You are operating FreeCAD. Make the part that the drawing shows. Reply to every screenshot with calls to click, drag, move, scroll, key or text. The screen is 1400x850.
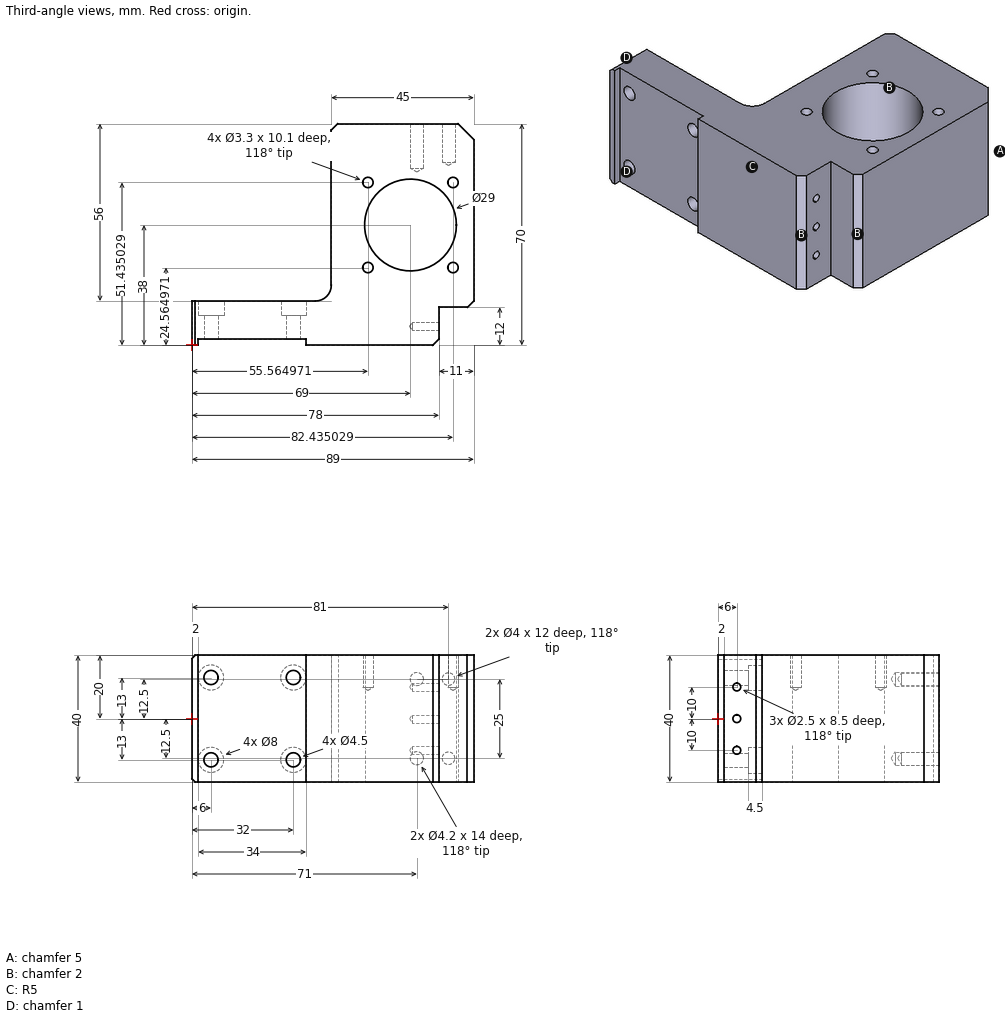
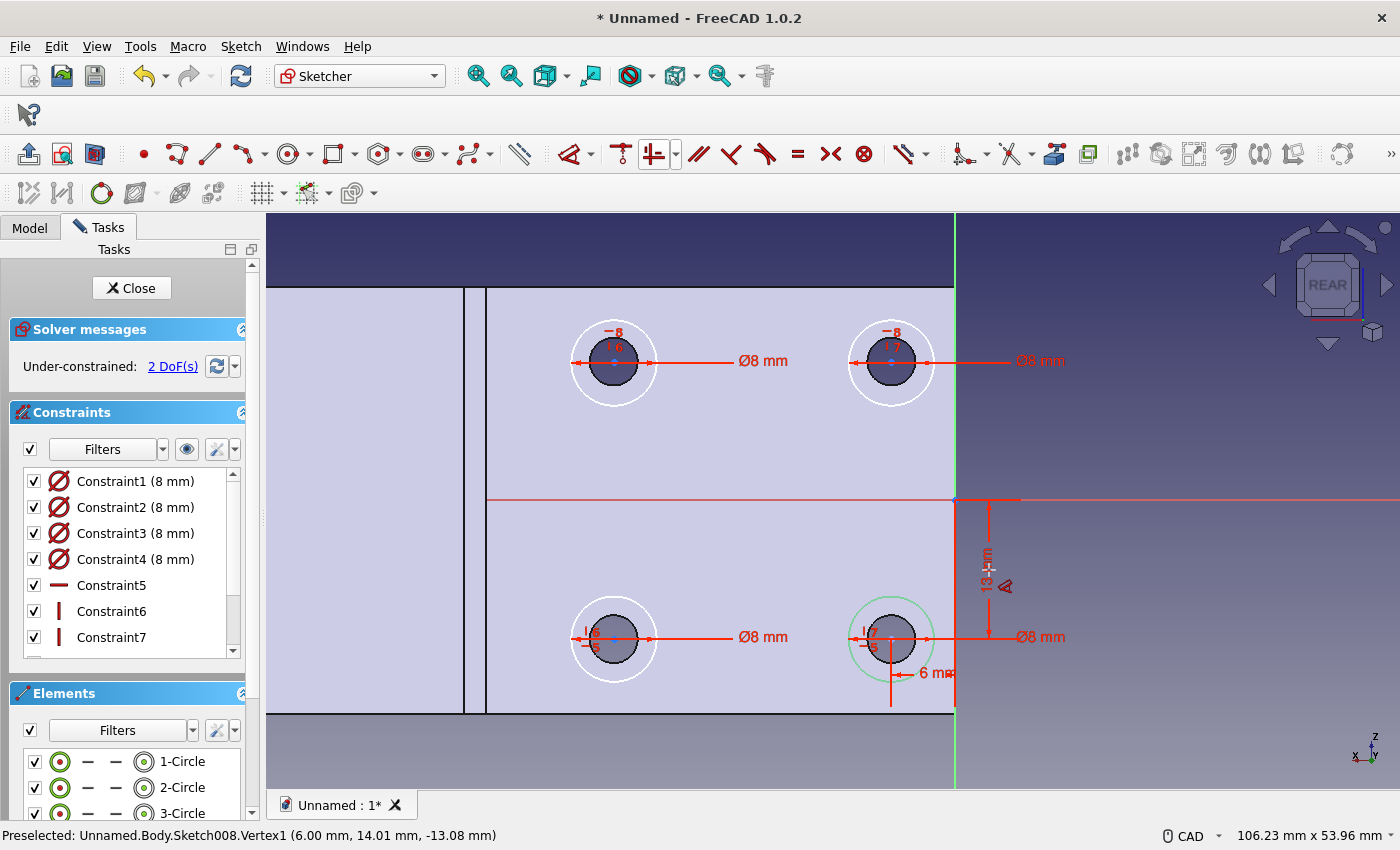
click(614, 639)
click(785, 673)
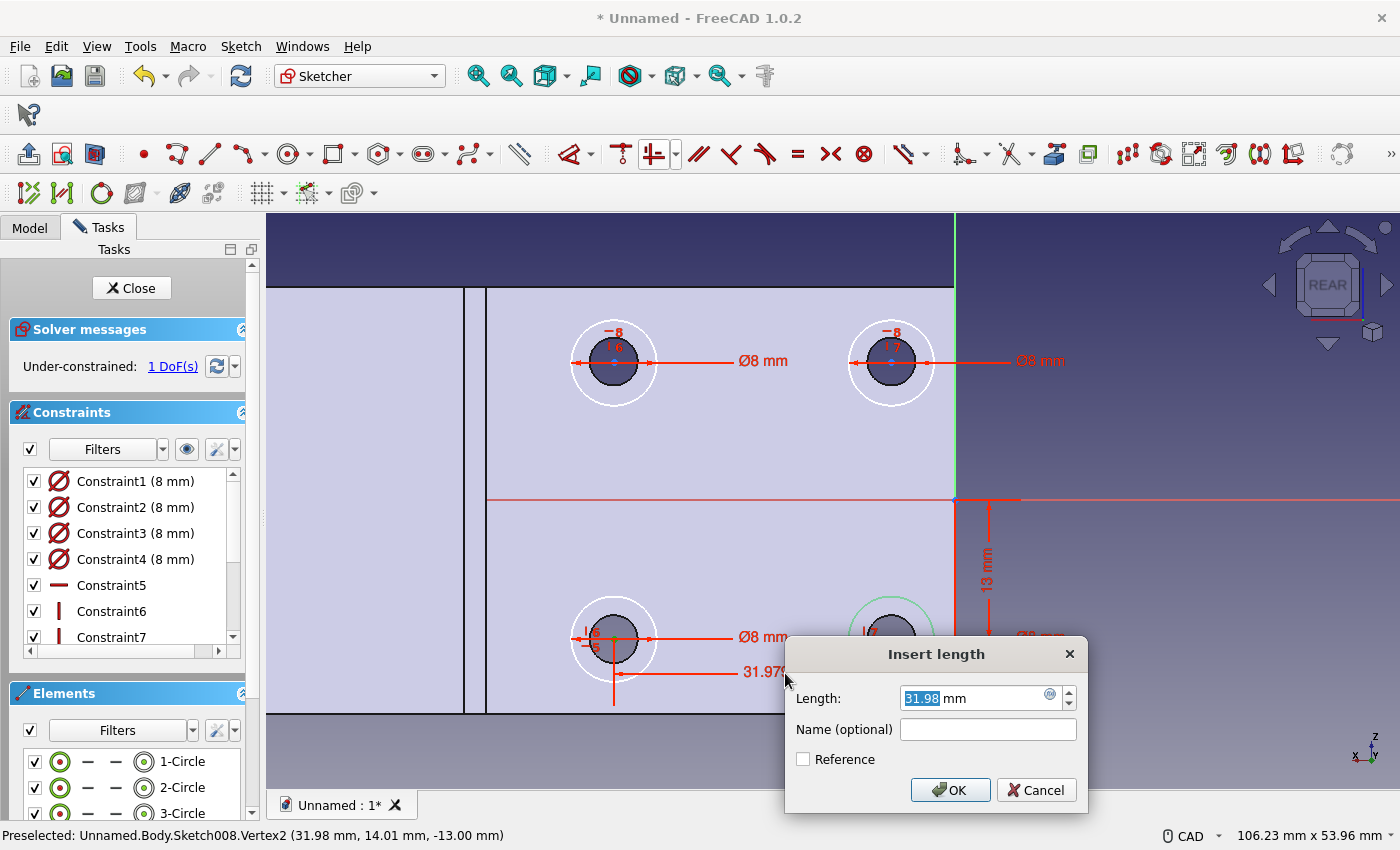
text(32)
key(Return)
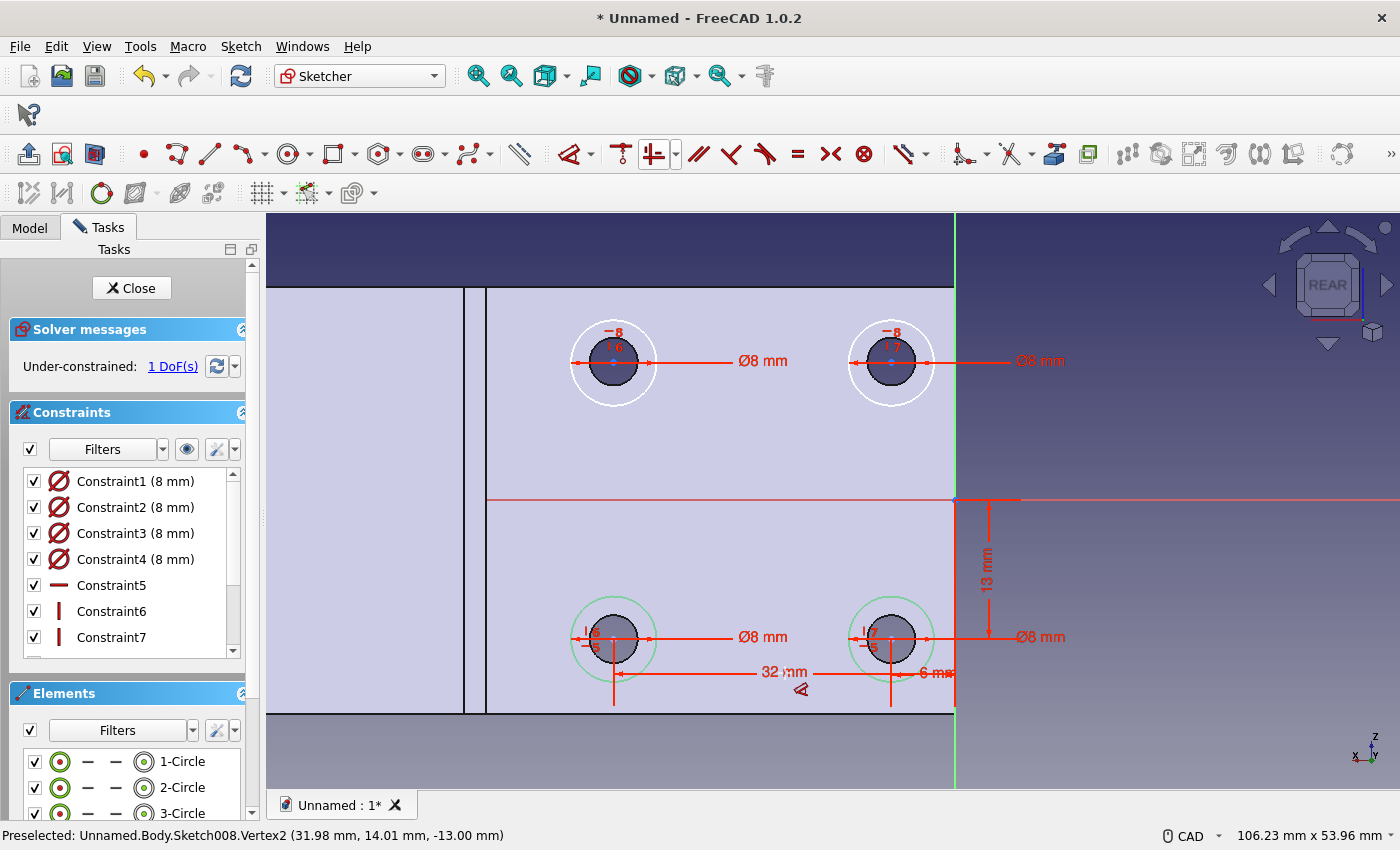
click(614, 363)
click(989, 432)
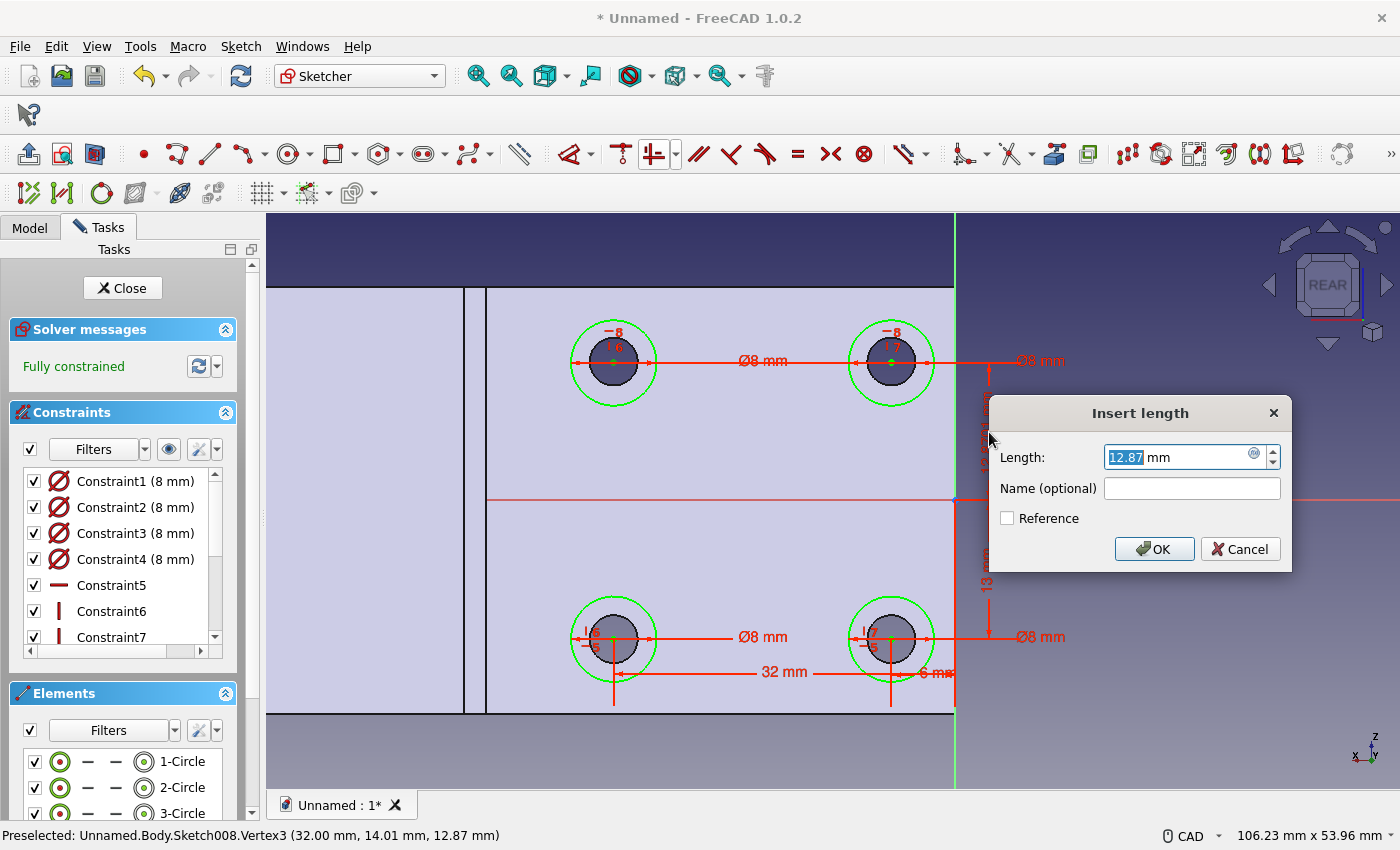
text(13)
key(Return)
key(Escape)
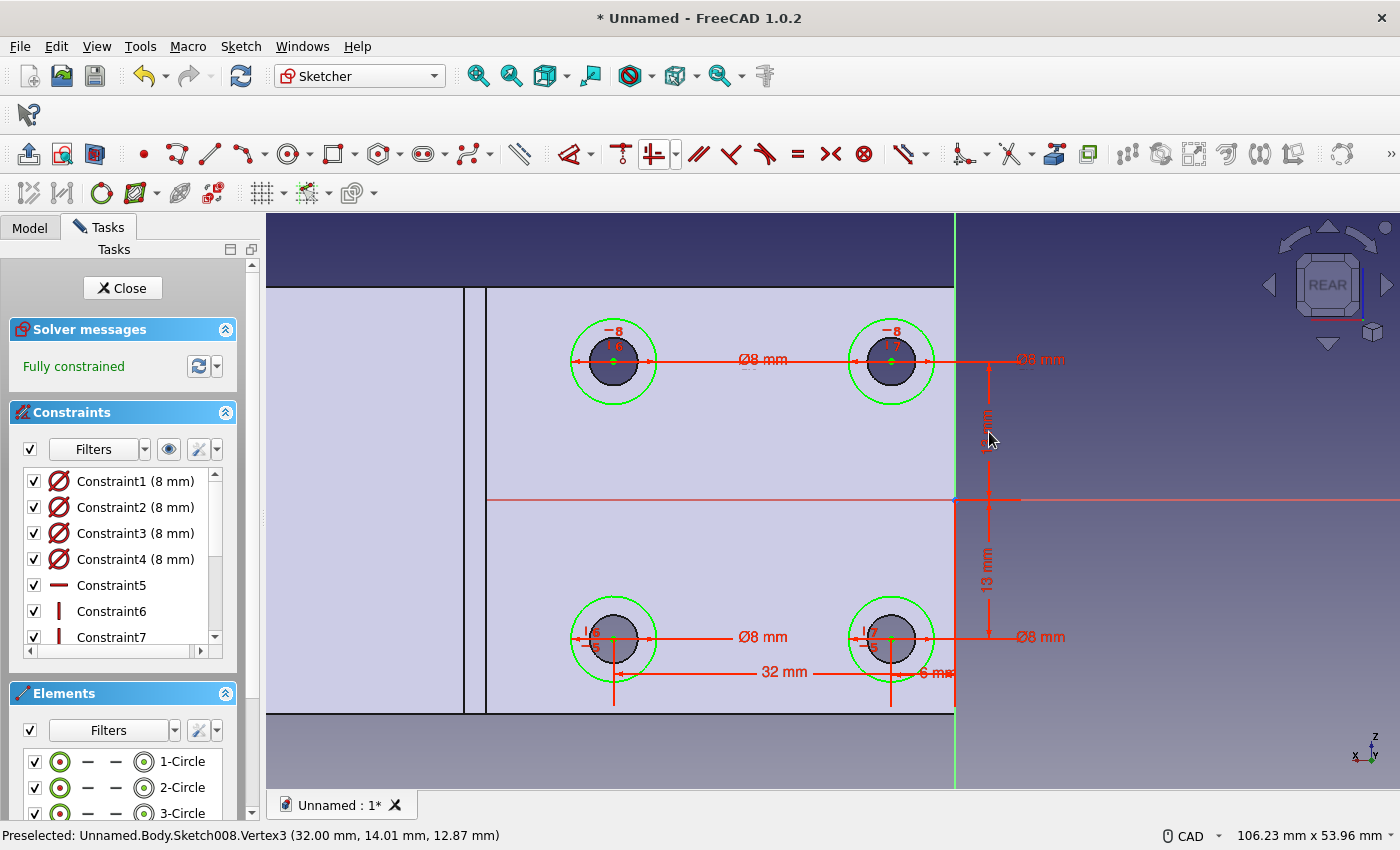
click(123, 288)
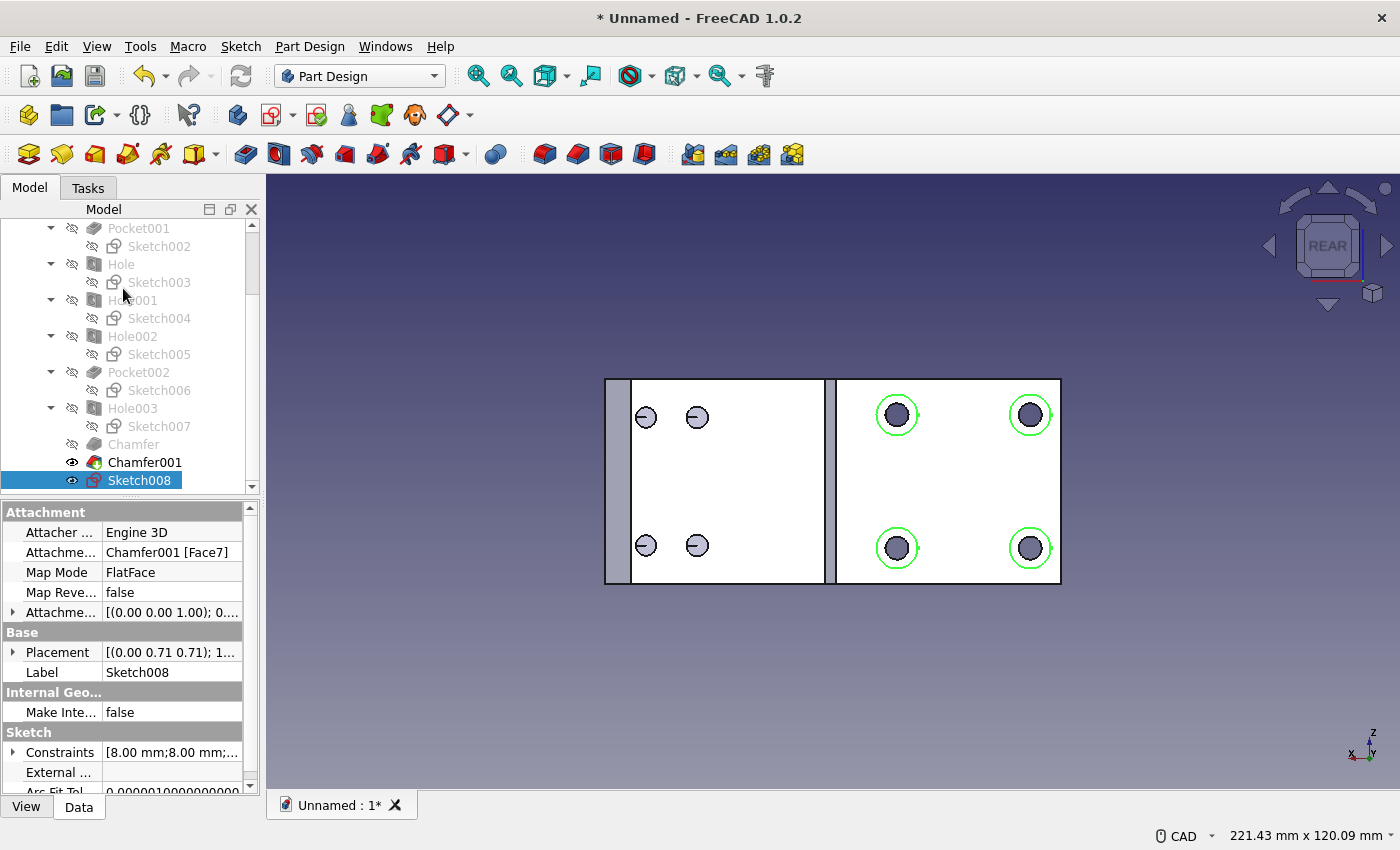
click(246, 154)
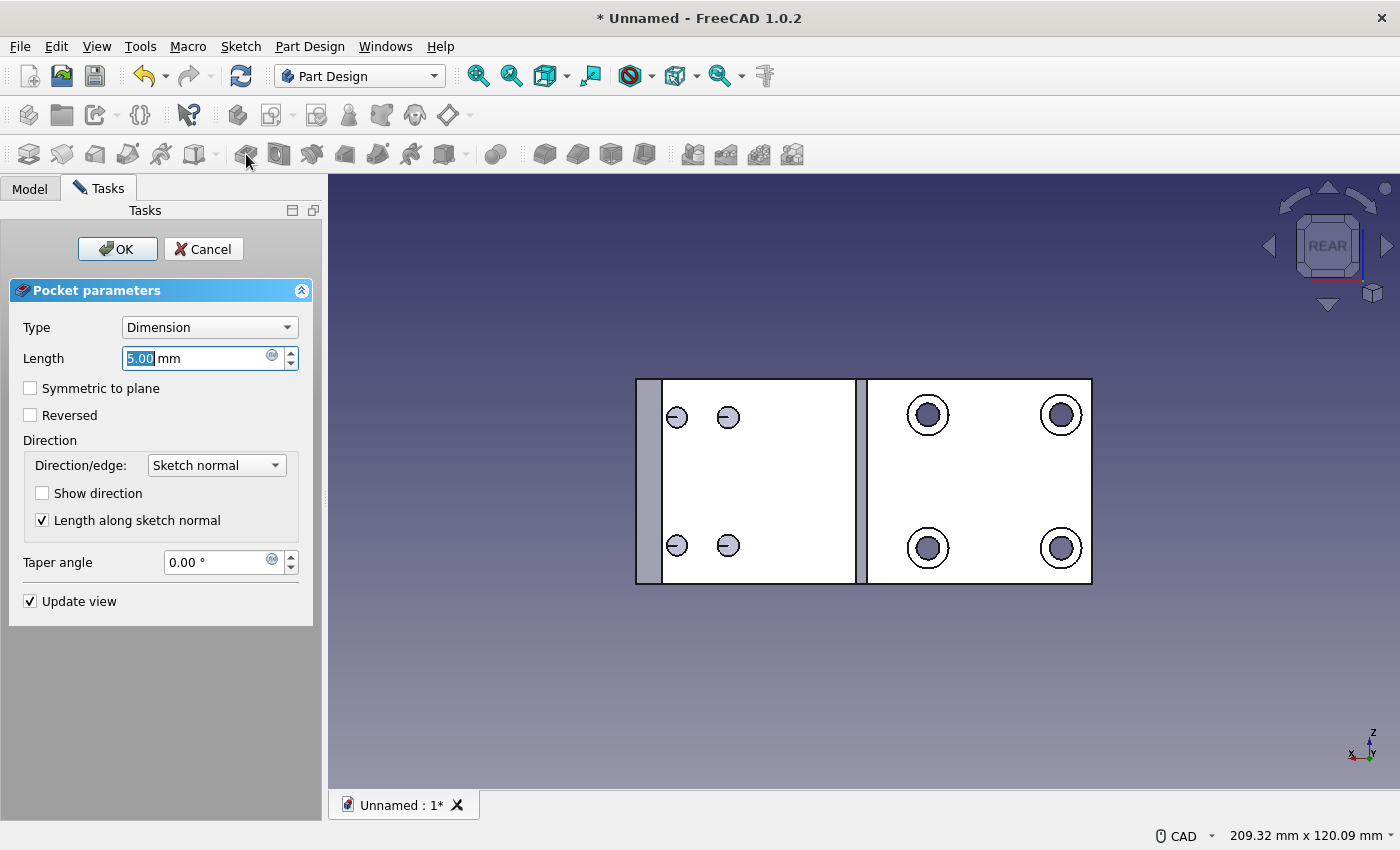
text(4.5)
key(Tab)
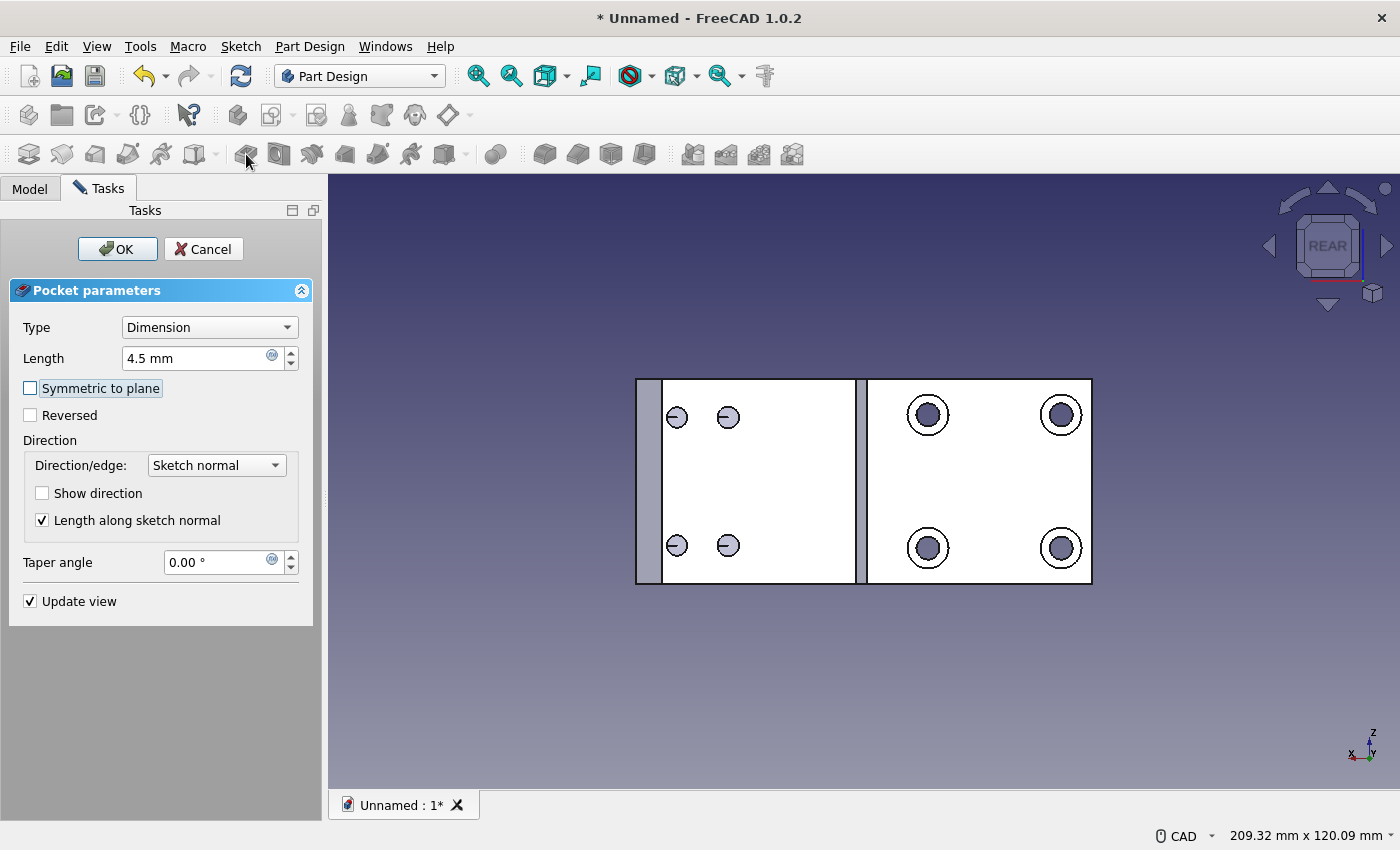
click(118, 249)